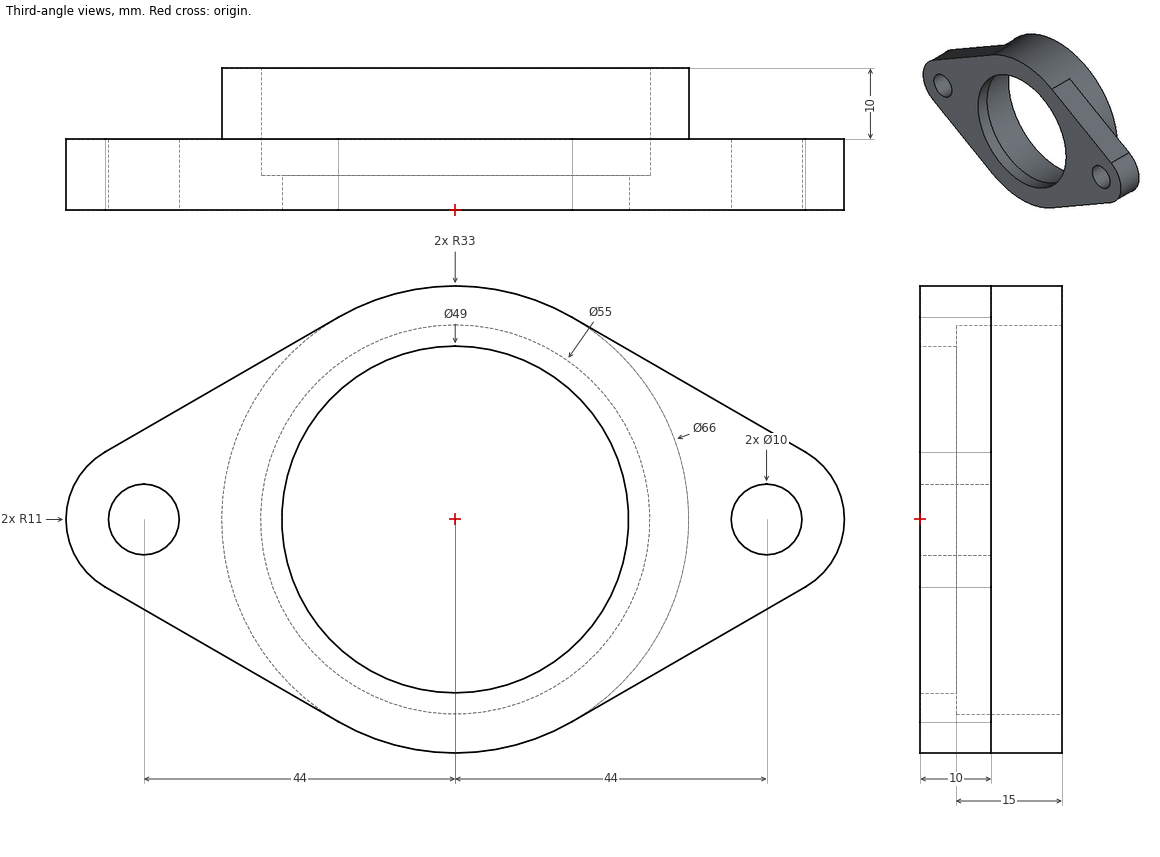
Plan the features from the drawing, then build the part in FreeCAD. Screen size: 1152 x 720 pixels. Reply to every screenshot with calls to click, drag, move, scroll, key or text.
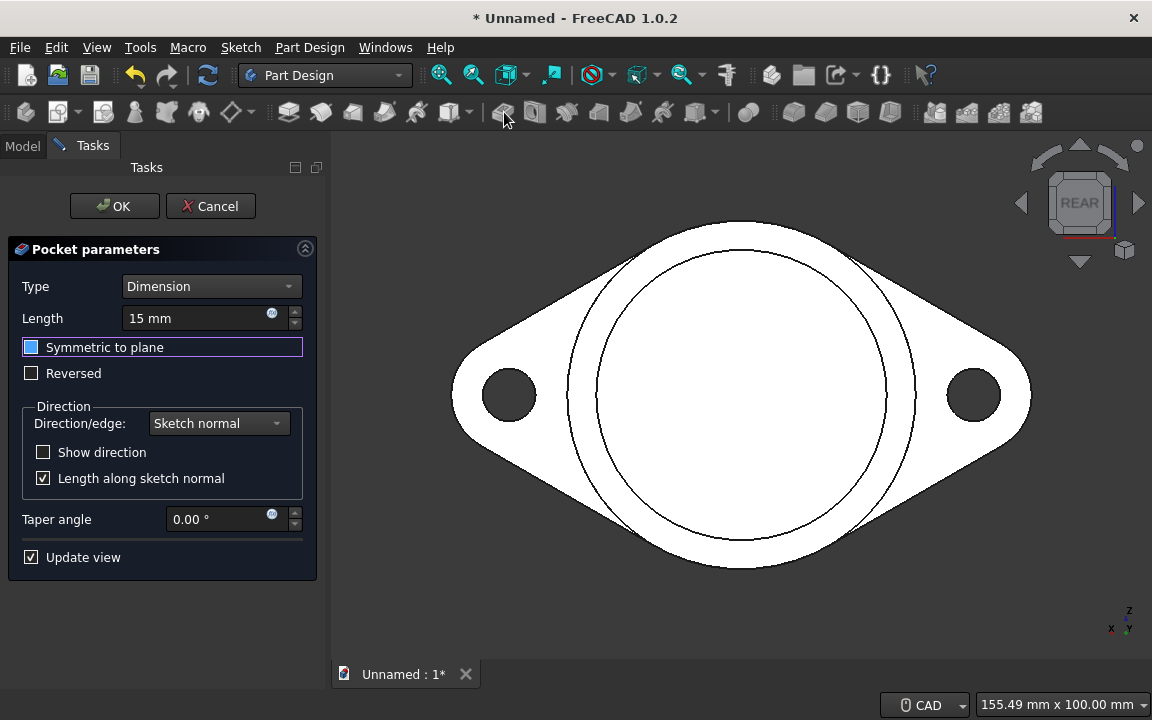
click(115, 206)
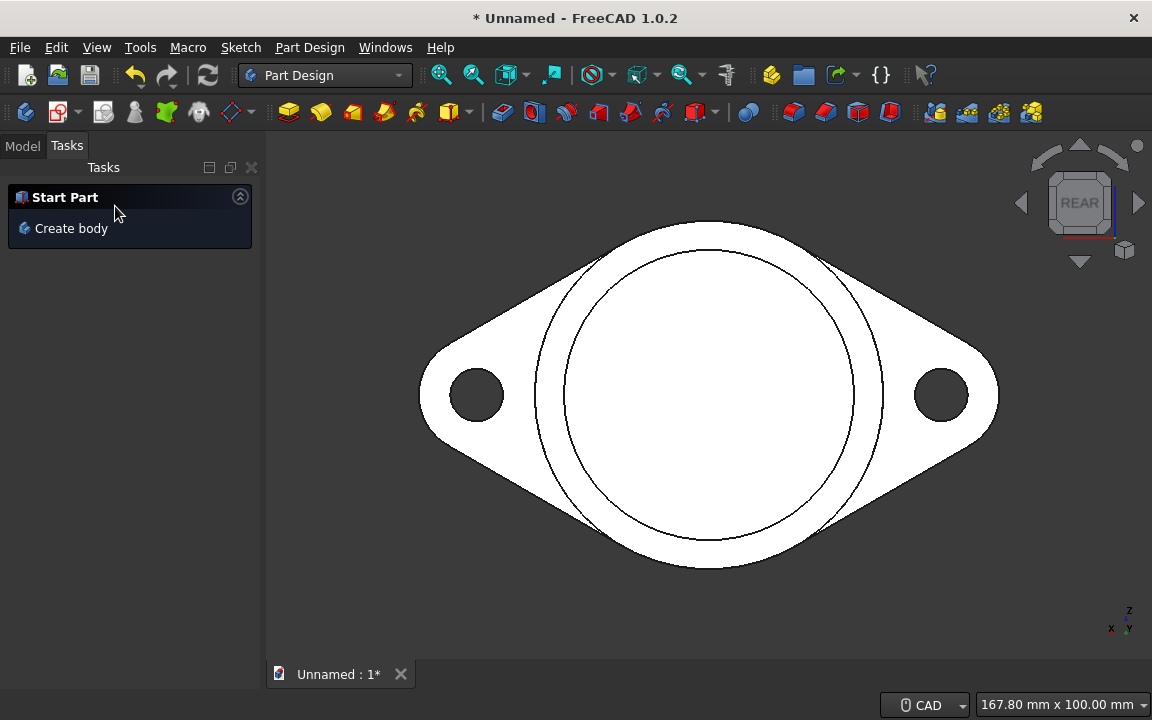
click(709, 394)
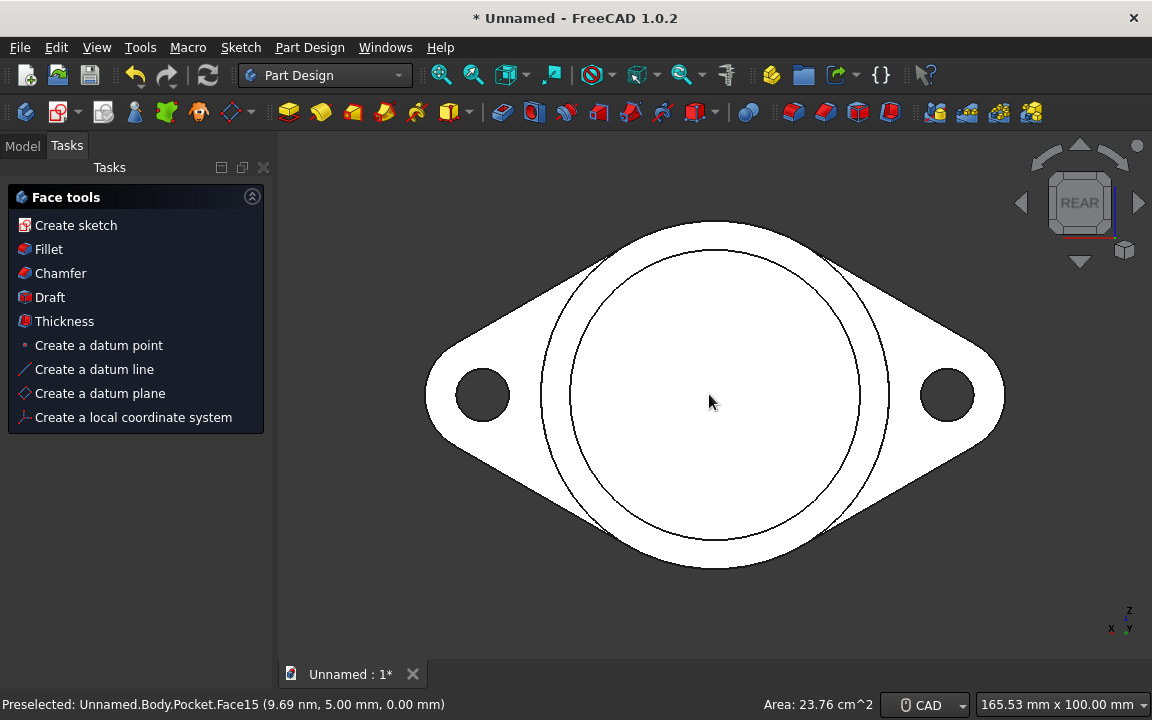
click(58, 112)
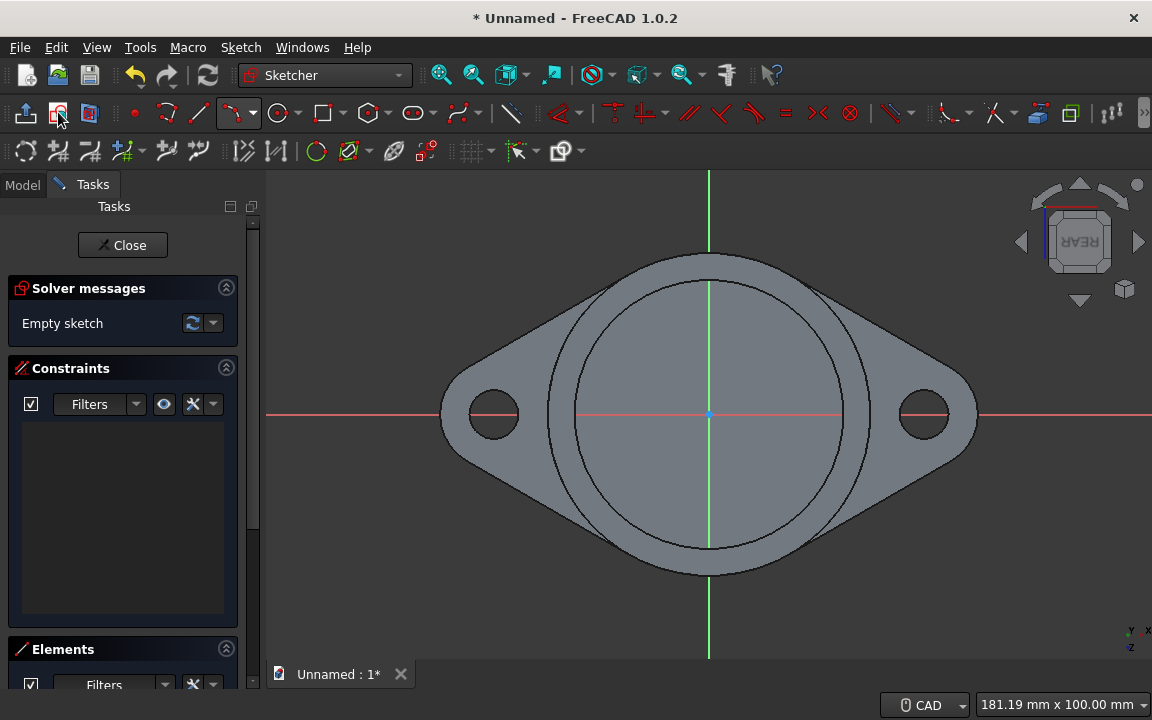
click(278, 114)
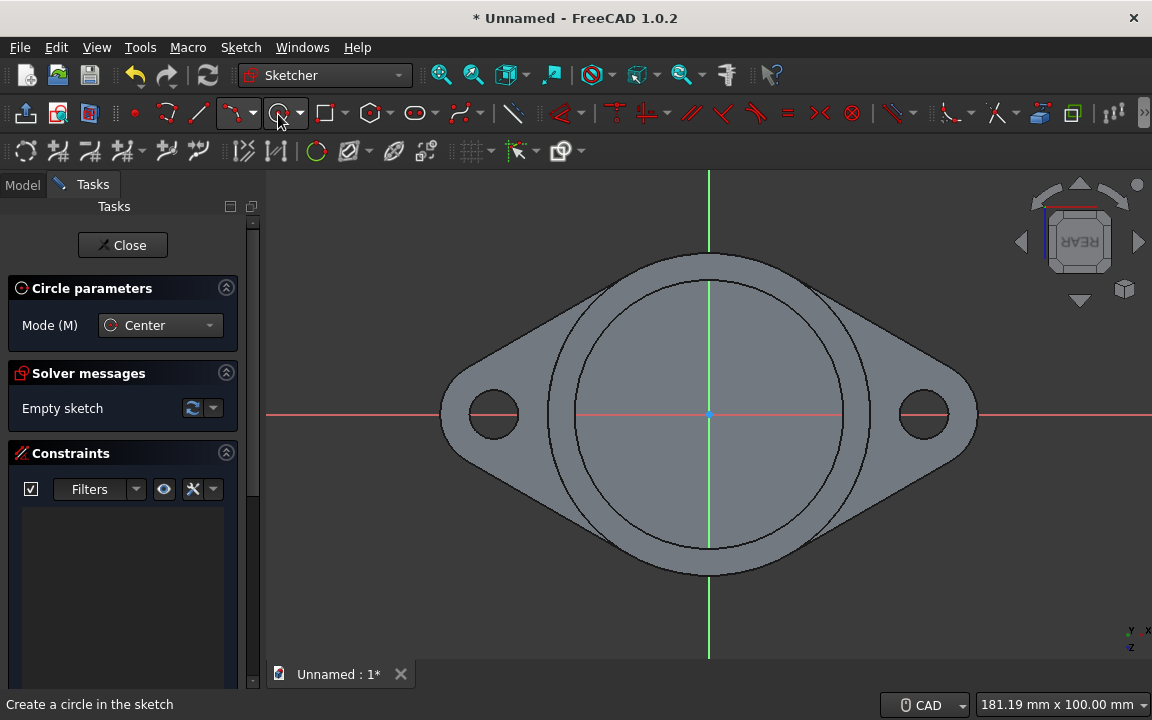
click(709, 414)
move(794, 330)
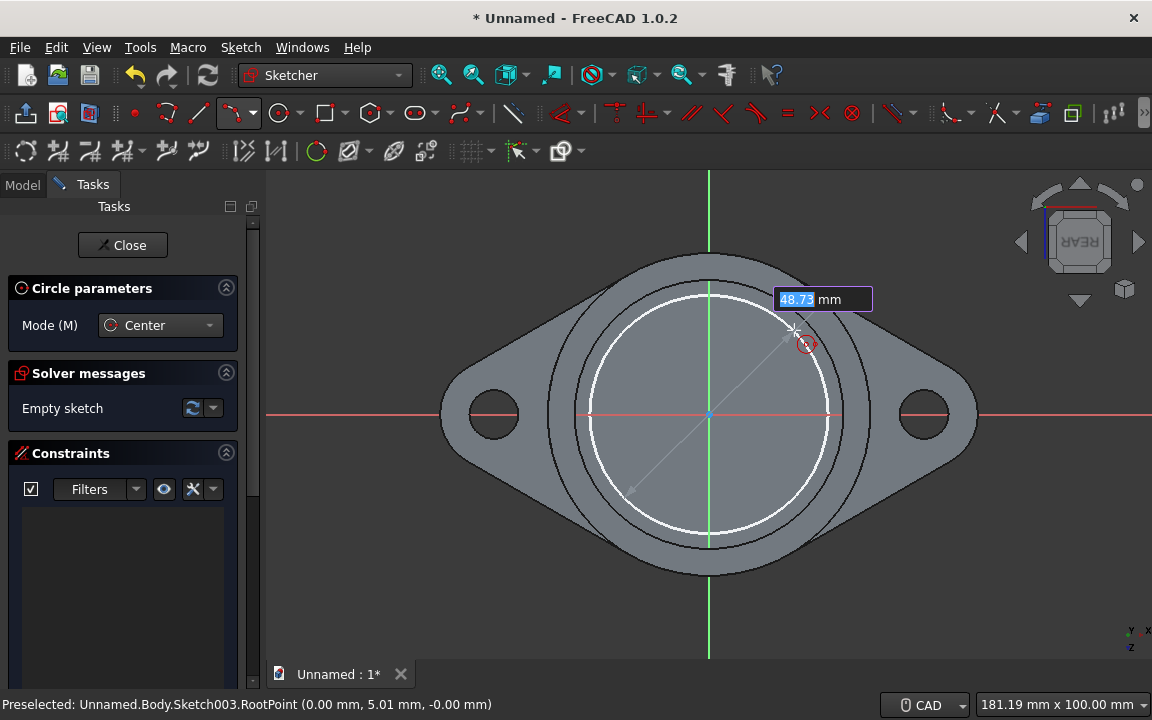
text(49)
key(Return)
key(Escape)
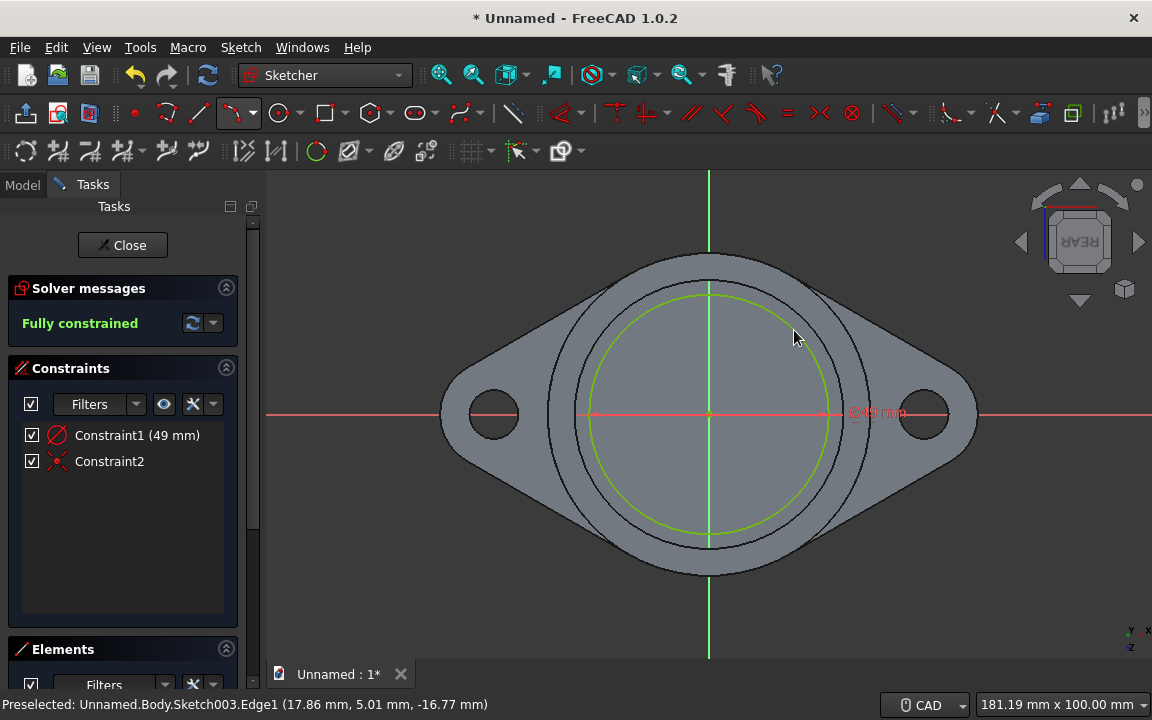
click(123, 245)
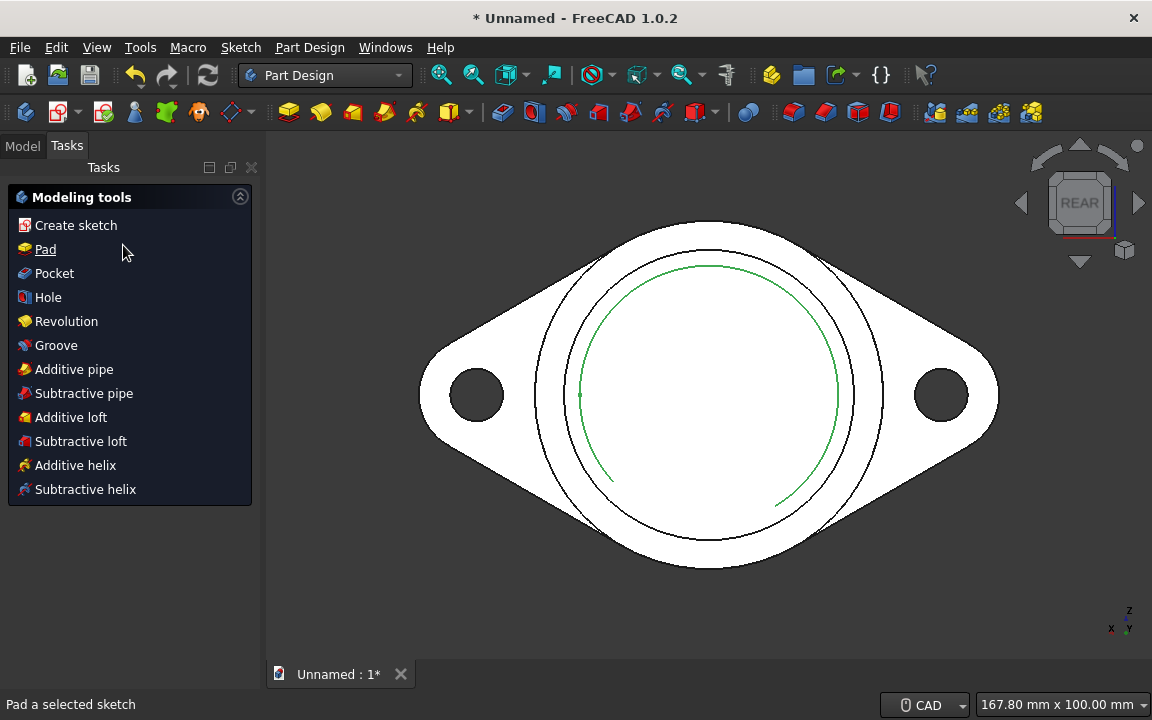
click(504, 112)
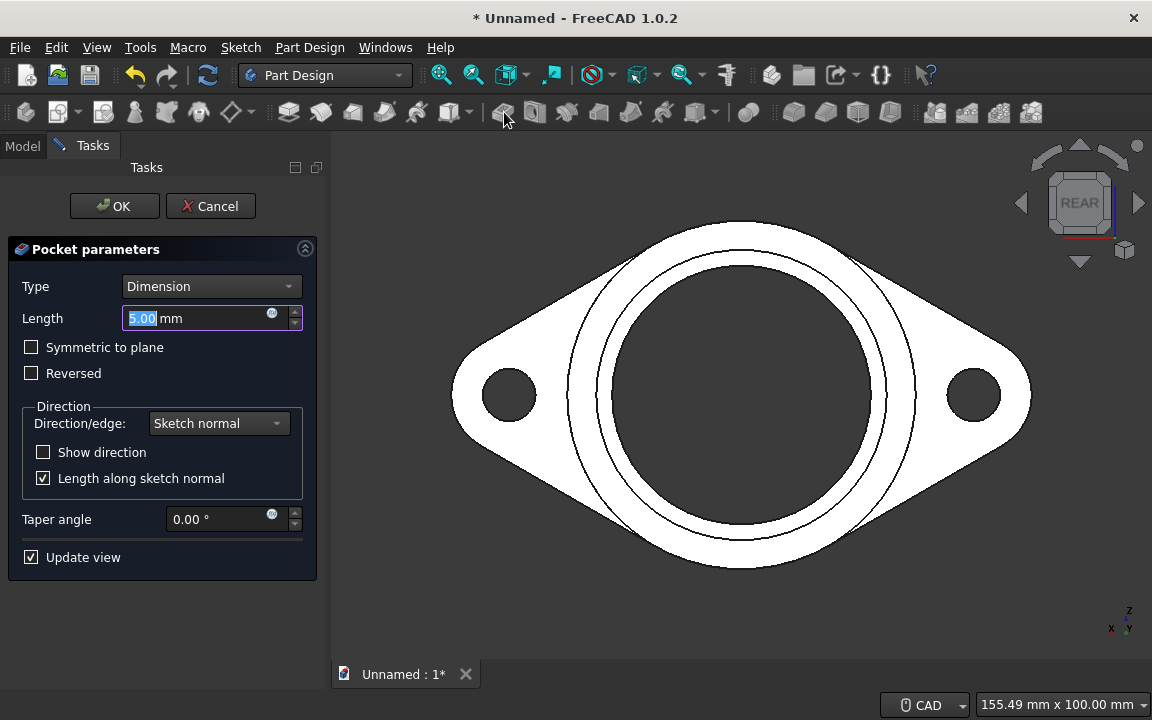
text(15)
key(Tab)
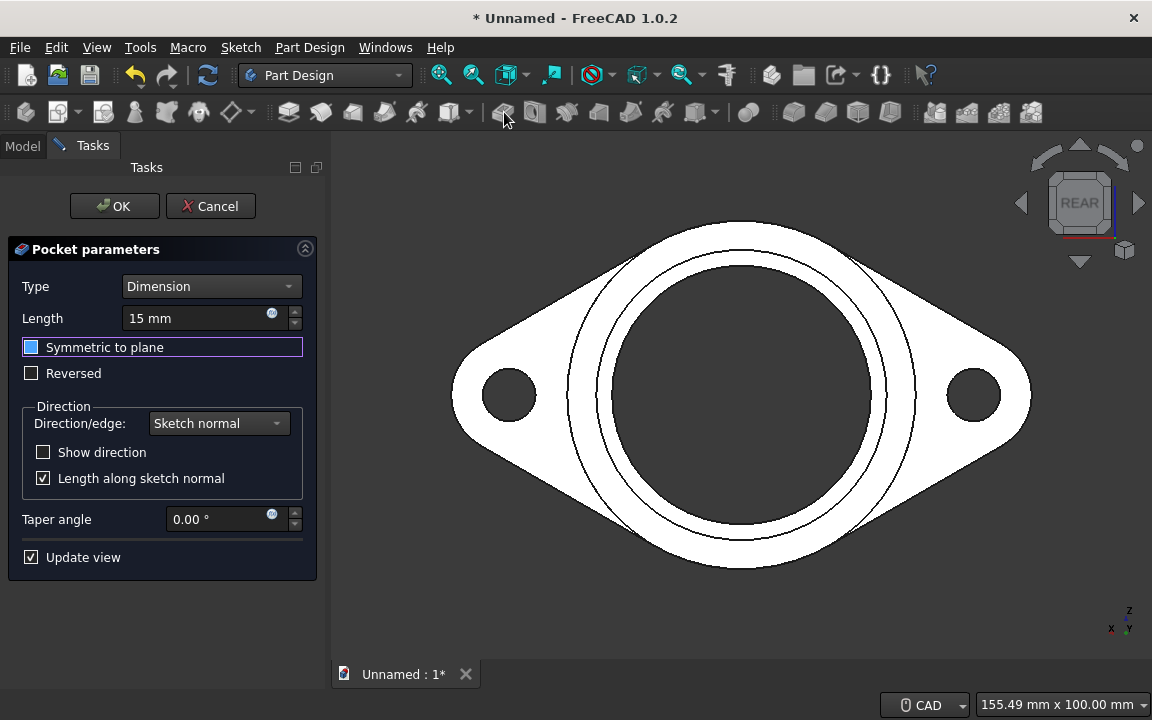
click(115, 206)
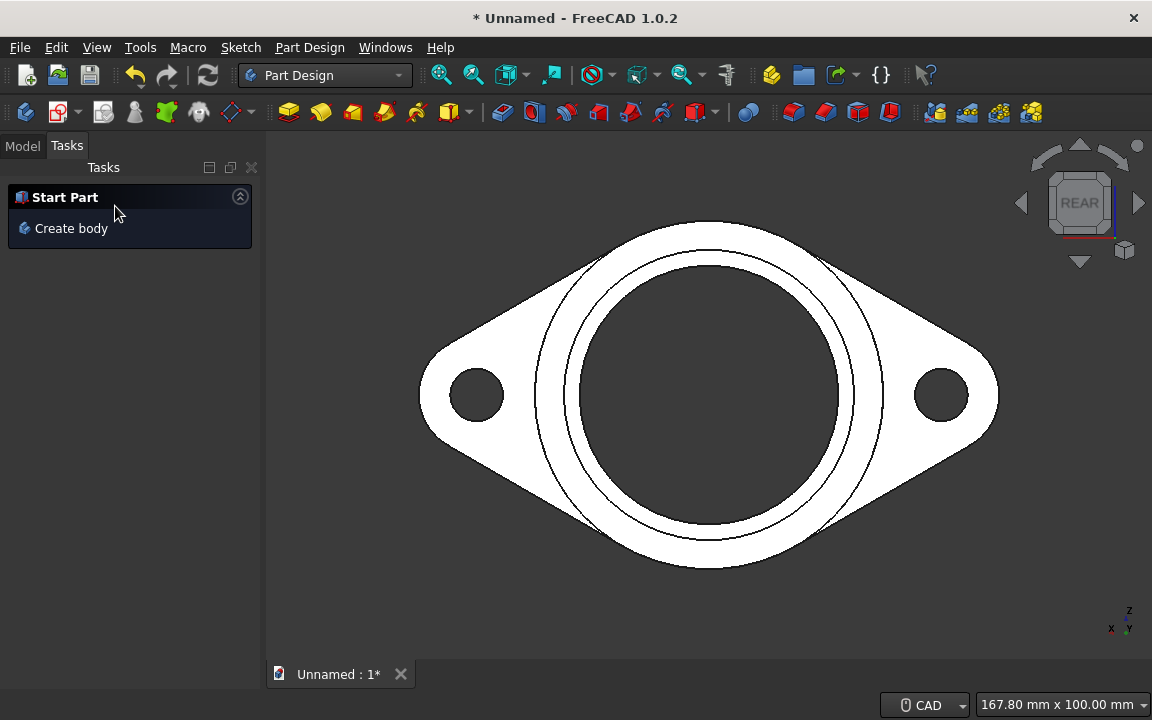
key(0)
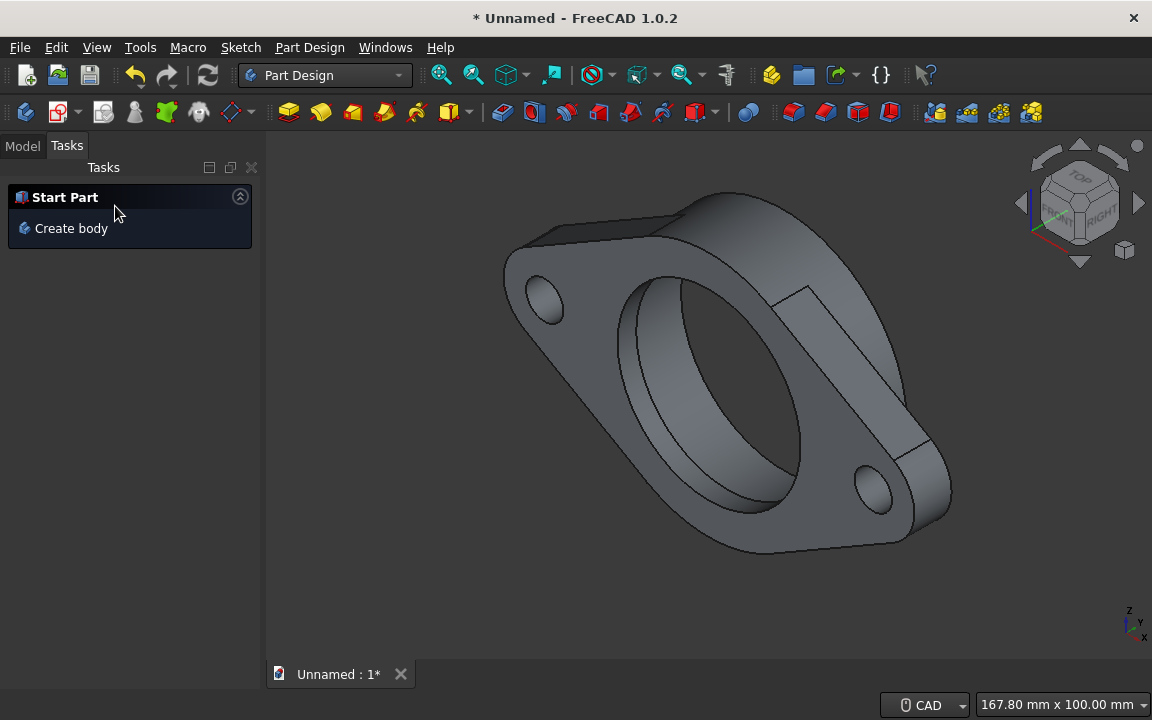
click(442, 76)